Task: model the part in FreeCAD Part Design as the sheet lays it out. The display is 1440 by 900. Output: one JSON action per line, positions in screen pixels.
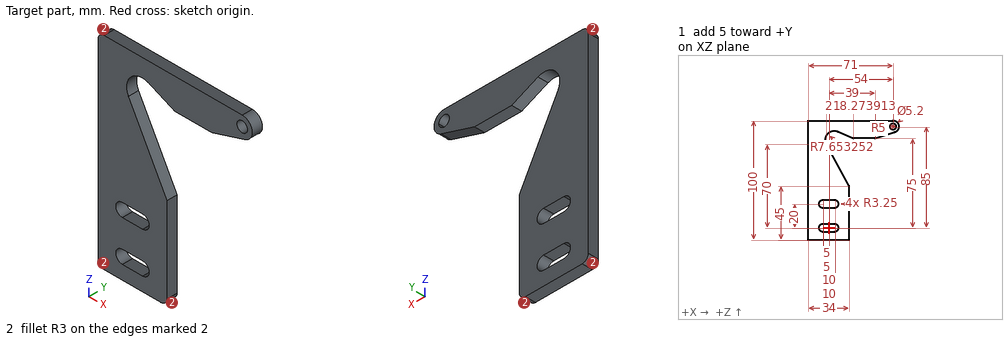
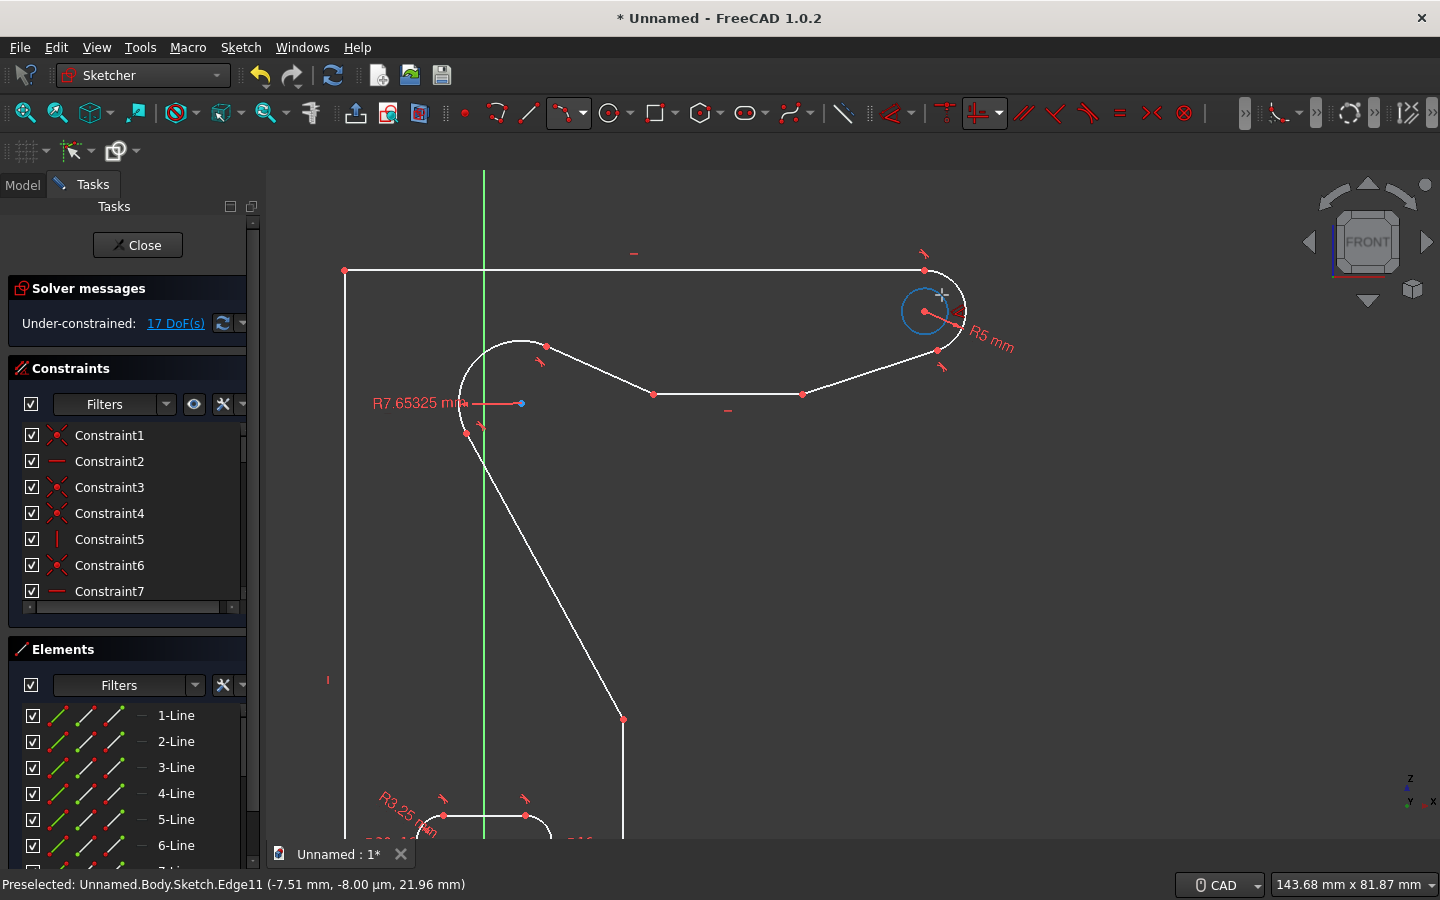
{"action": "left_click", "coordinate": [941, 295]}
{"action": "left_click", "coordinate": [963, 272]}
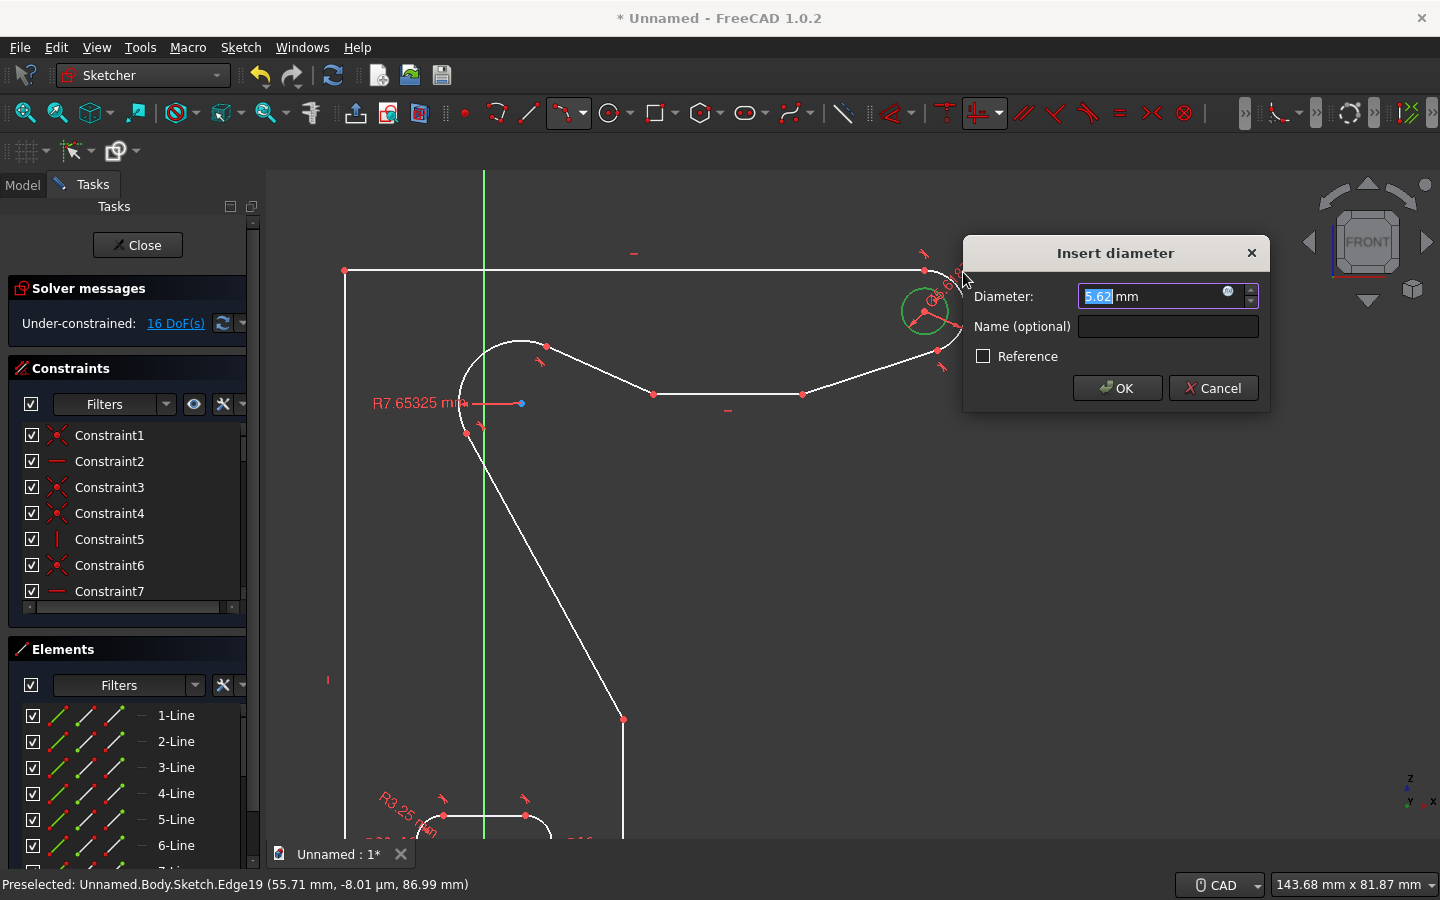
{"action": "type", "text": "5.2"}
{"action": "key", "text": "Return"}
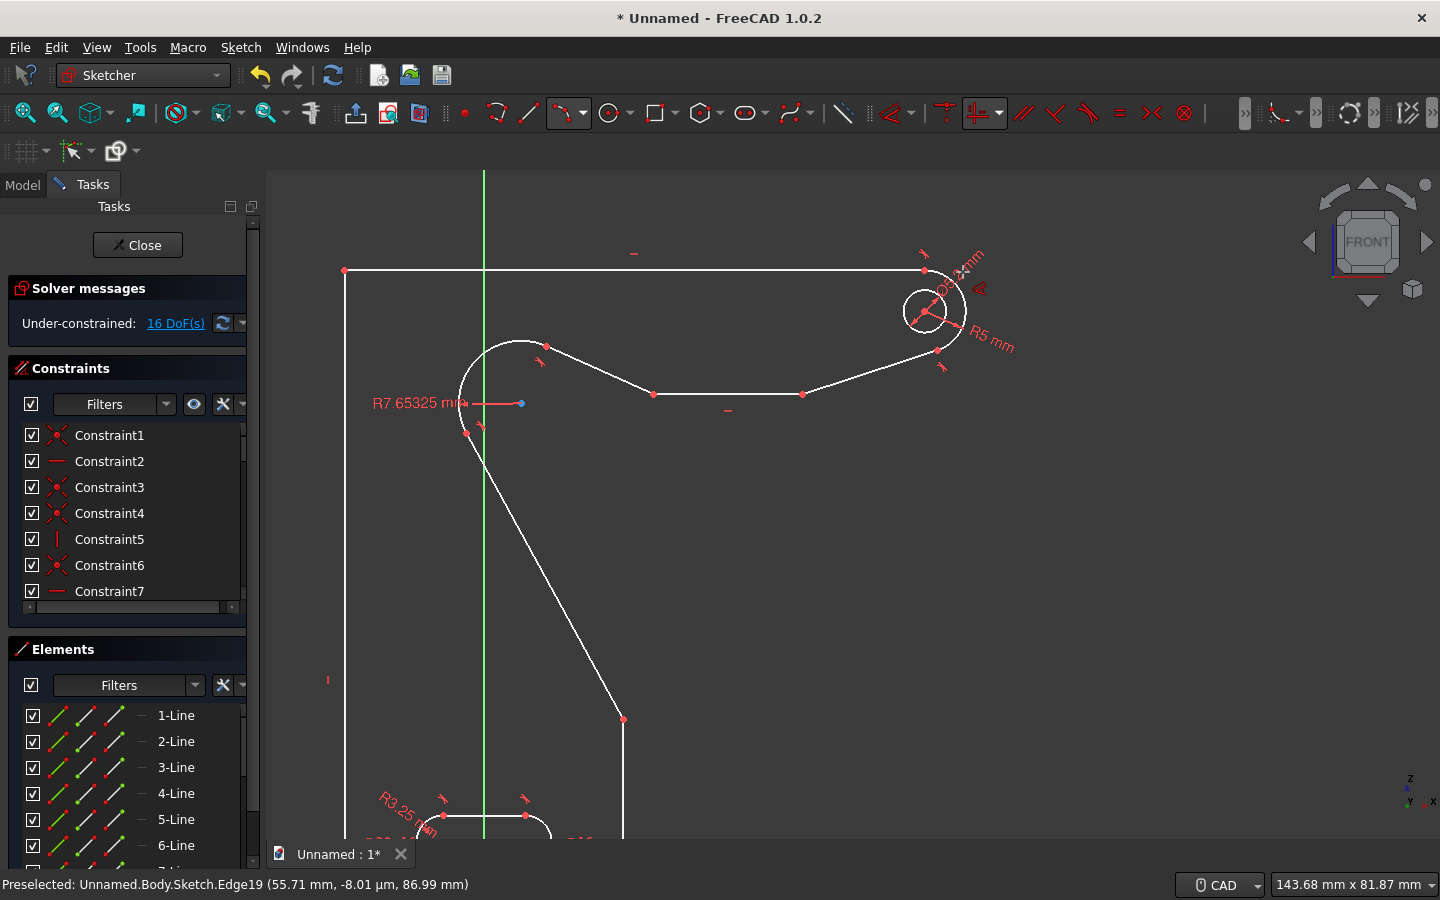
{"action": "left_click", "coordinate": [623, 793]}
{"action": "left_click", "coordinate": [589, 765]}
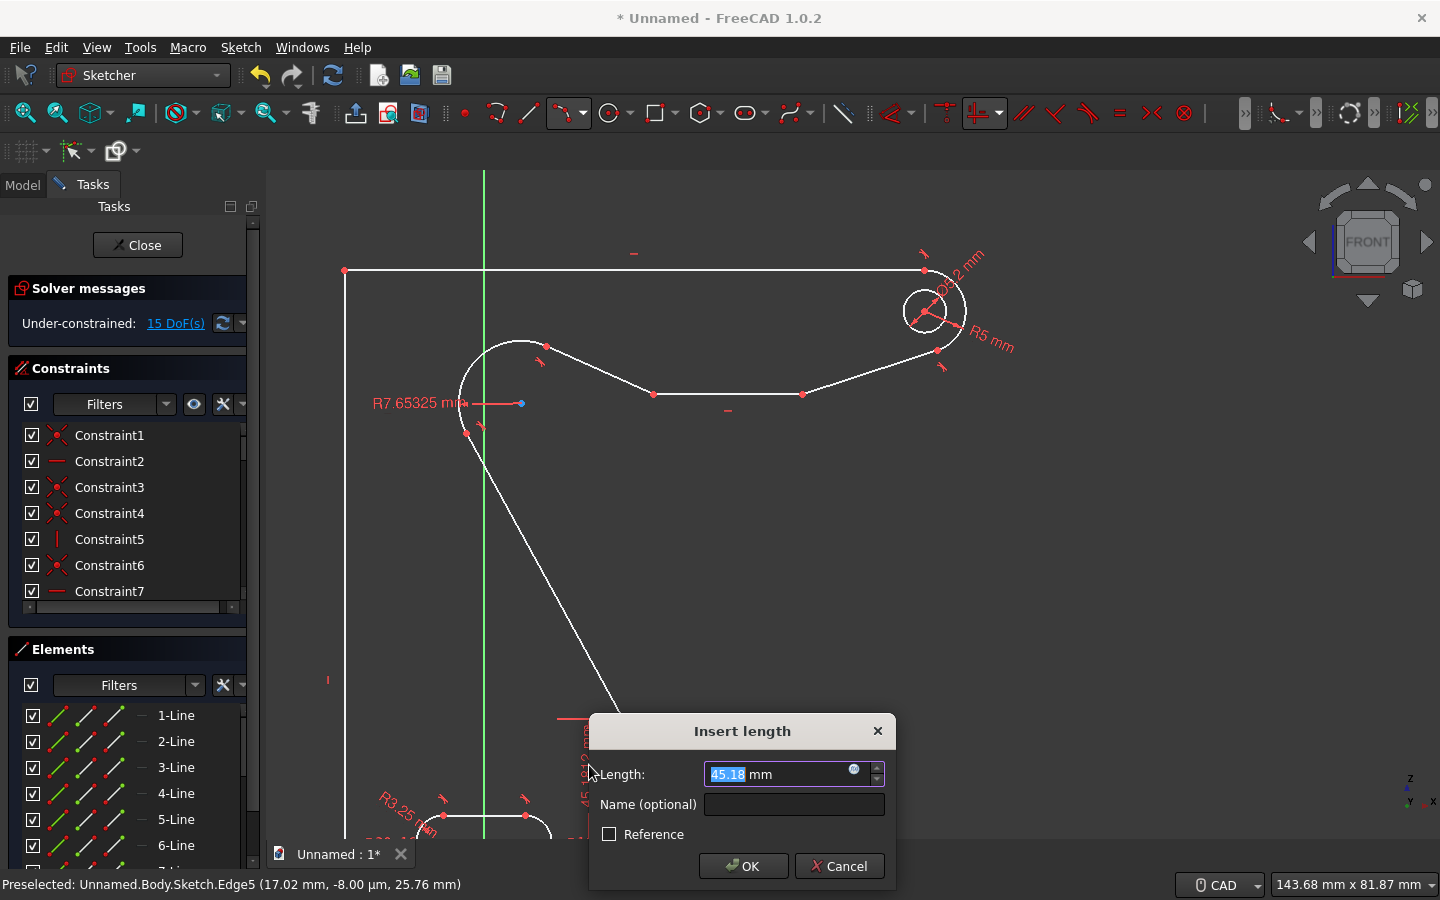
{"action": "type", "text": "45"}
{"action": "key", "text": "Return"}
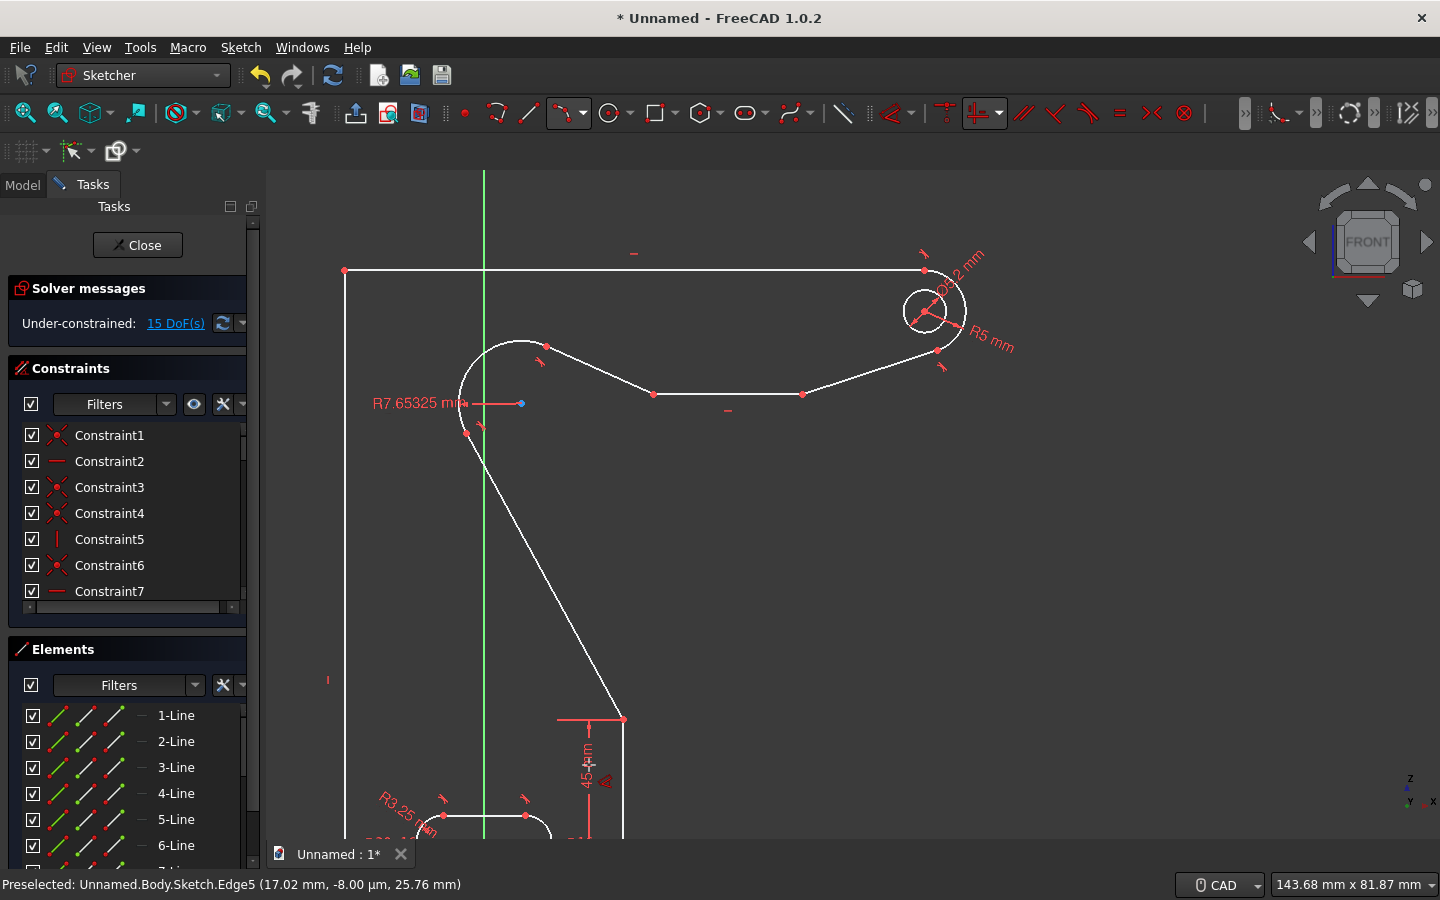
{"action": "scroll", "coordinate": [941, 294], "scroll_direction": "down", "scroll_amount": 3}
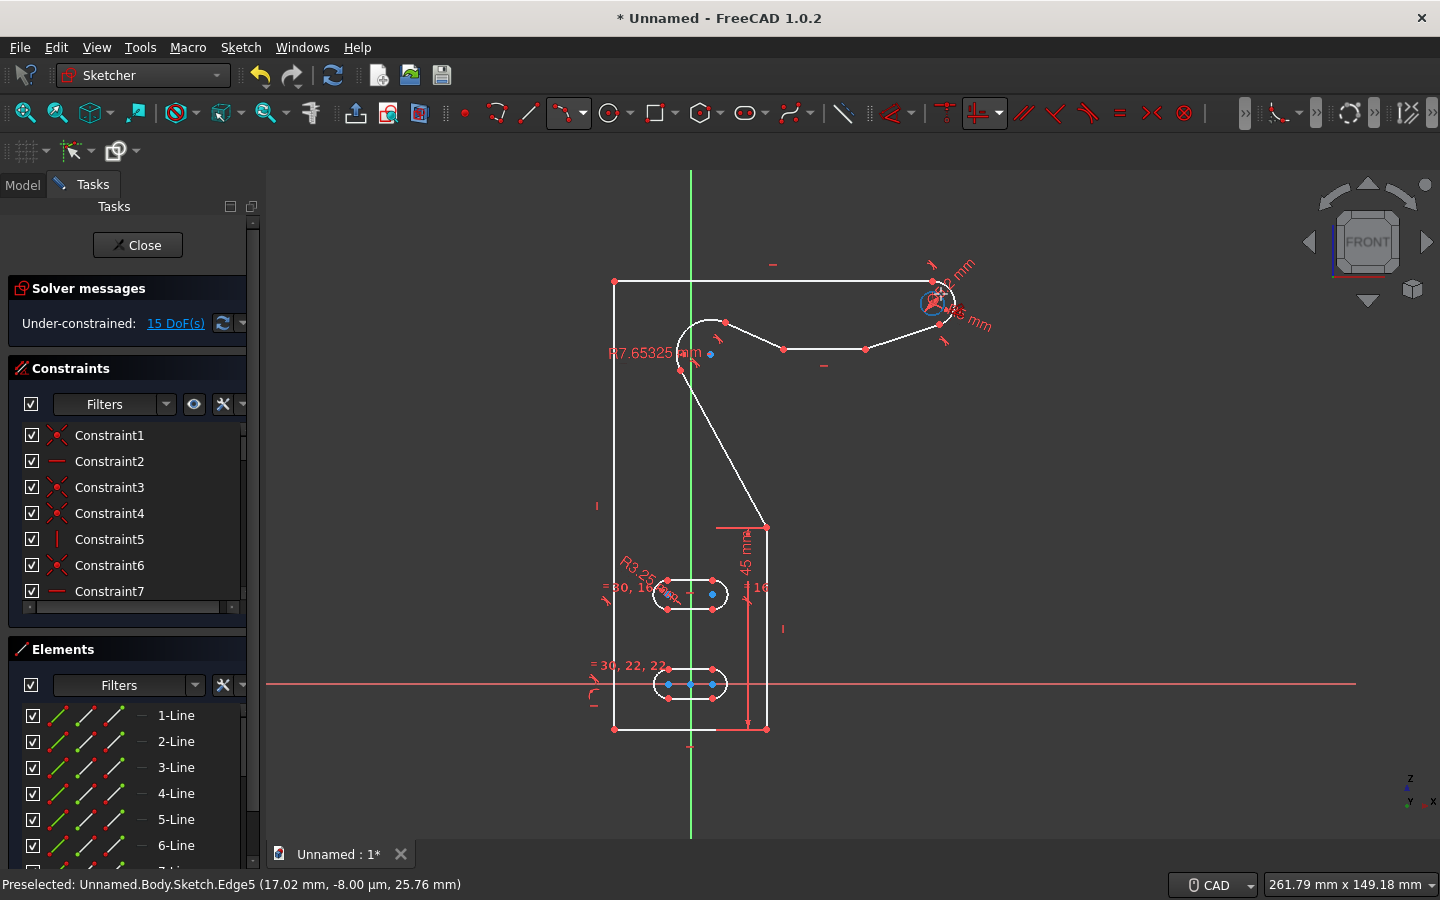
{"action": "left_click", "coordinate": [721, 730]}
{"action": "left_click", "coordinate": [655, 764]}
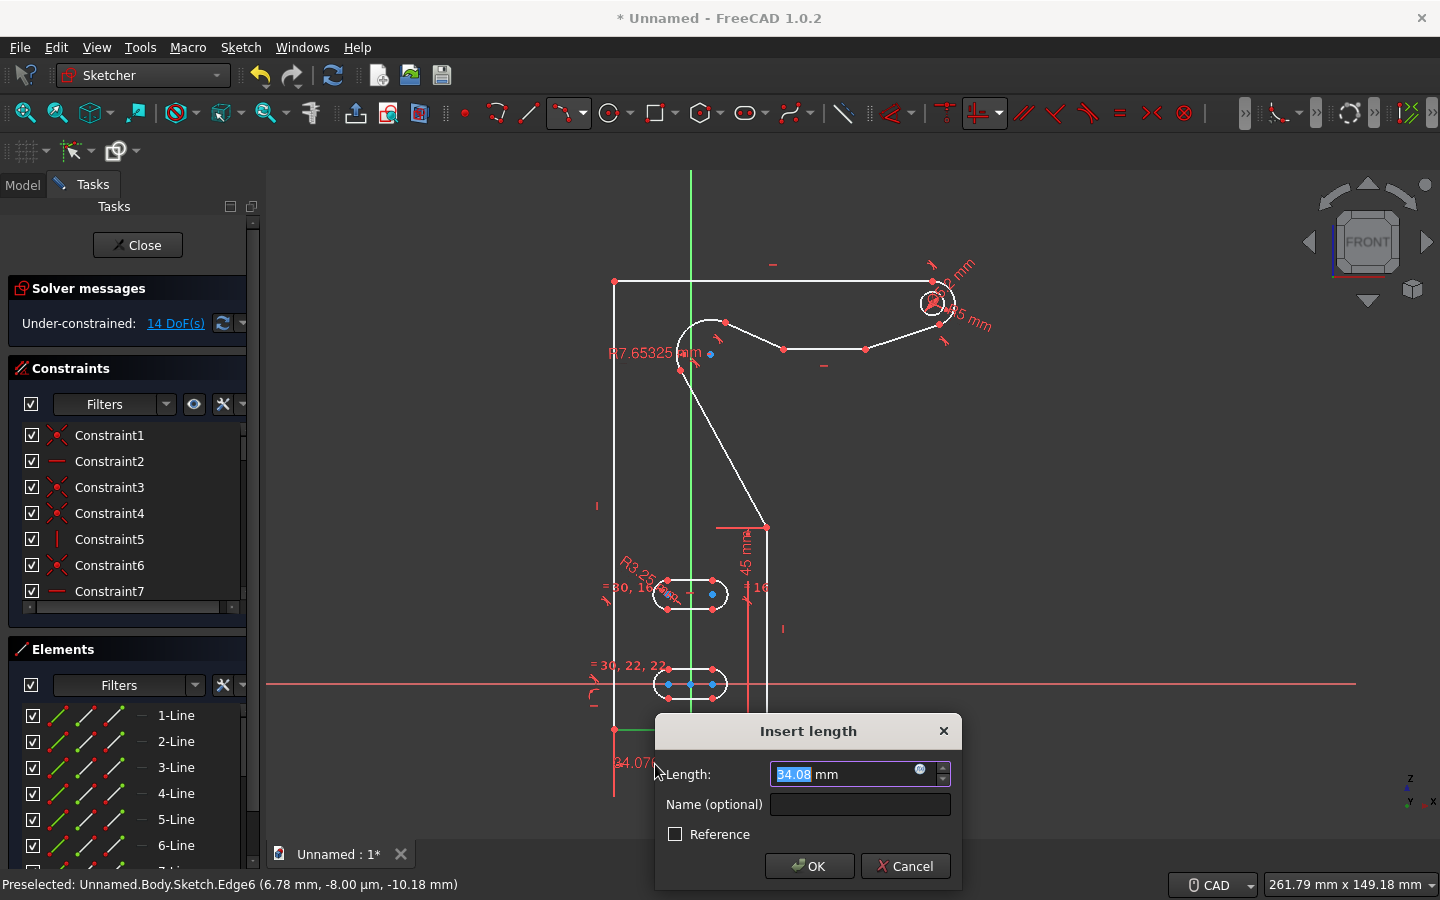
{"action": "type", "text": "34"}
{"action": "key", "text": "Return"}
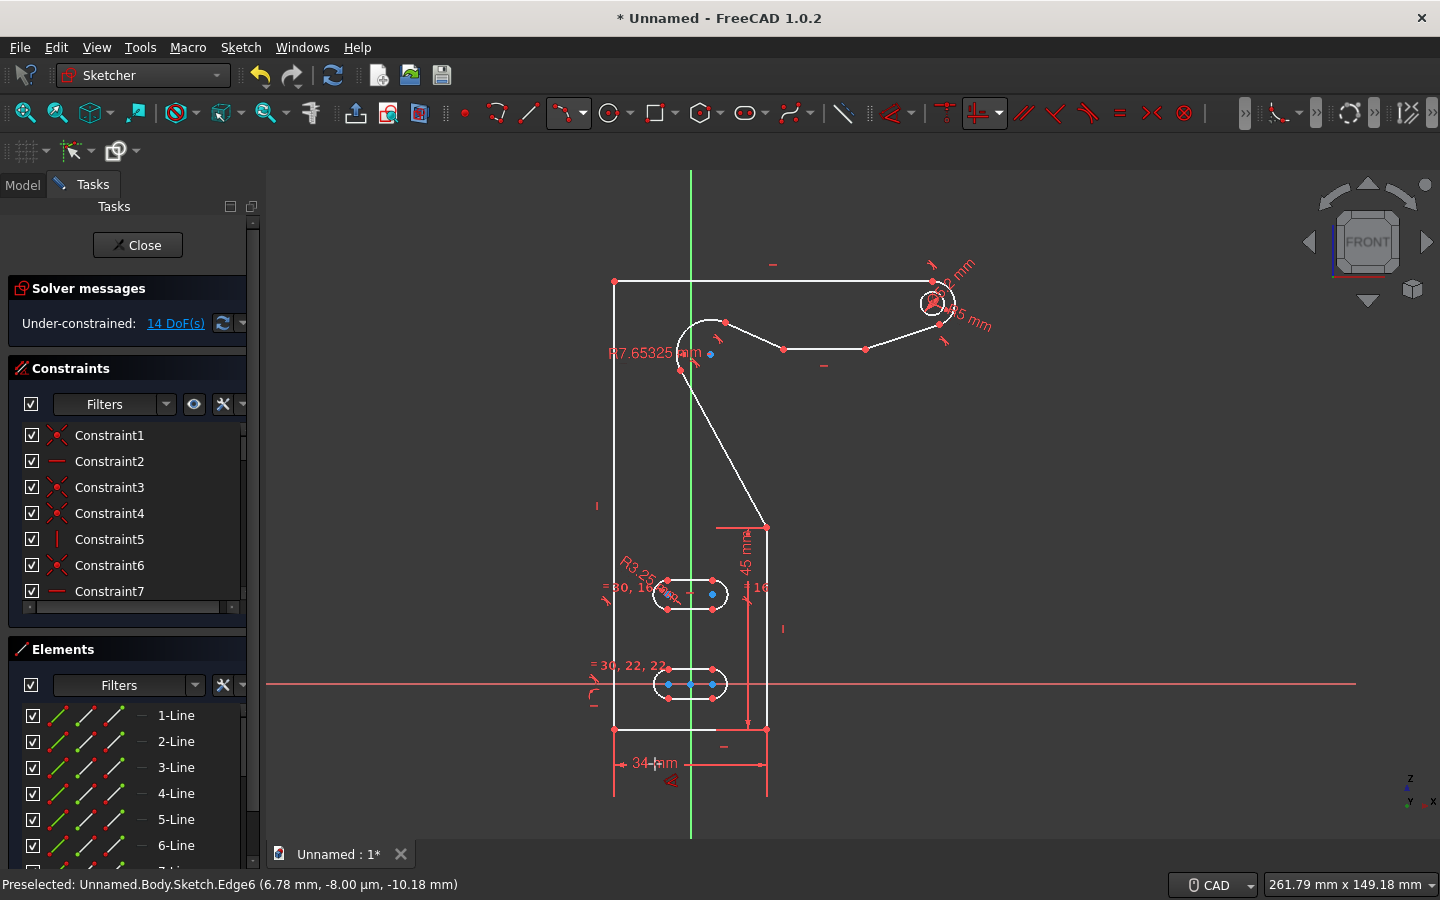
{"action": "left_click", "coordinate": [710, 281]}
{"action": "left_click", "coordinate": [773, 247]}